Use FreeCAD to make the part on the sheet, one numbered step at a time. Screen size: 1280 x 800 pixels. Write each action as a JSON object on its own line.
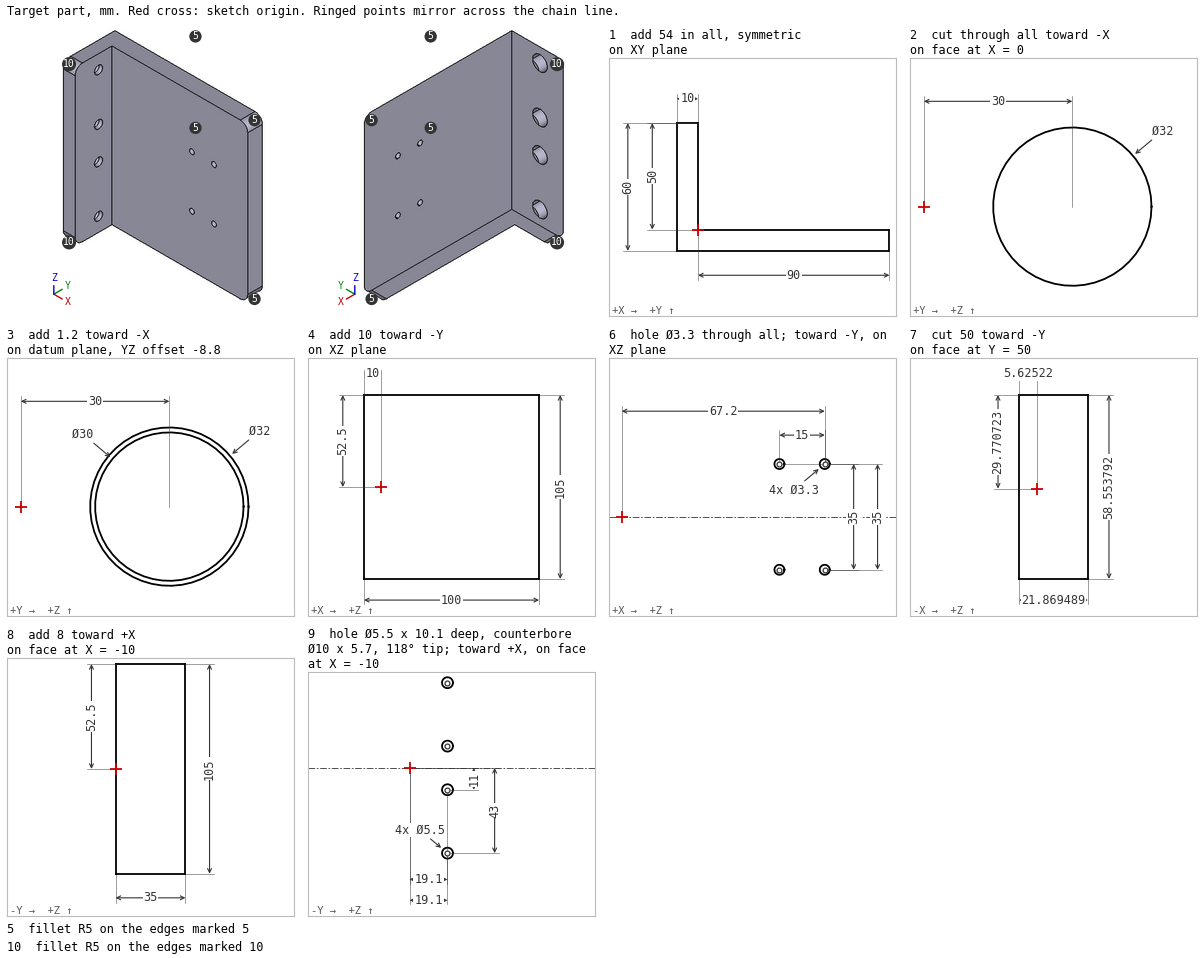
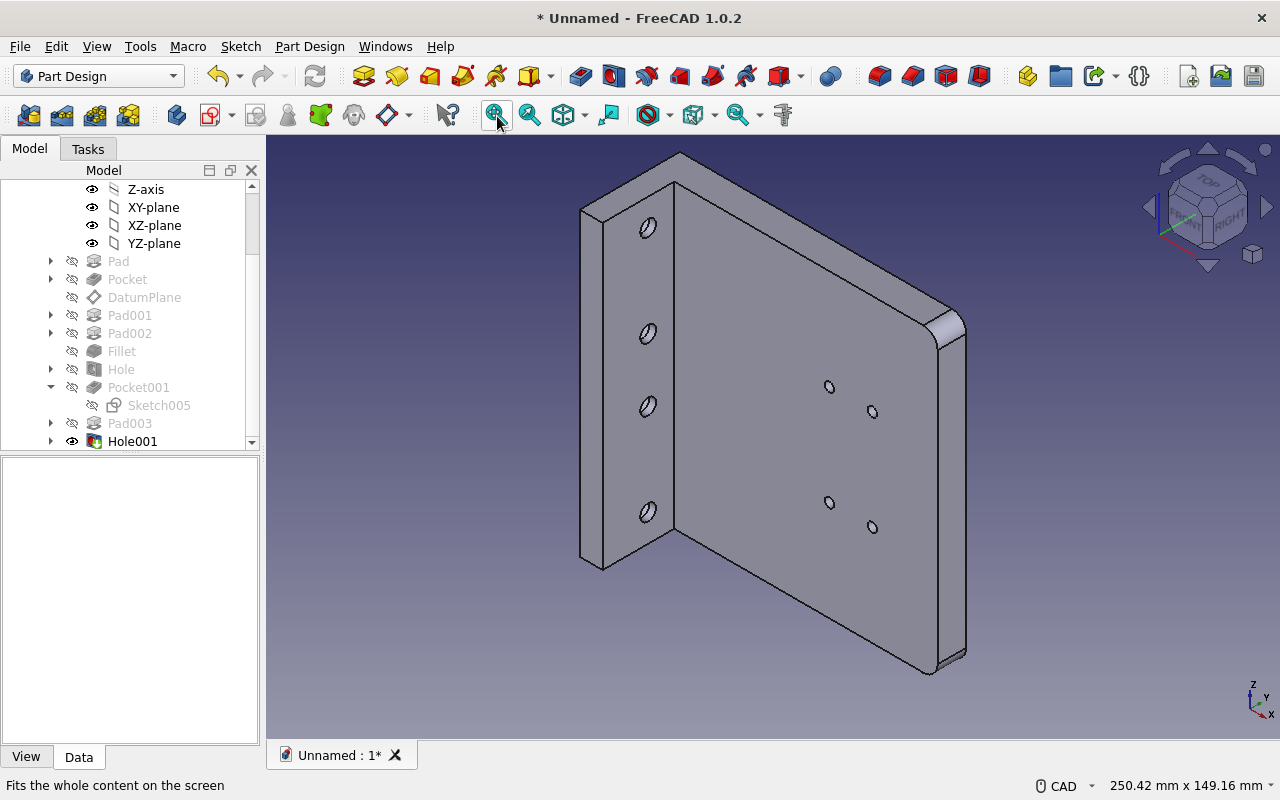
{"action": "left_click", "coordinate": [591, 215]}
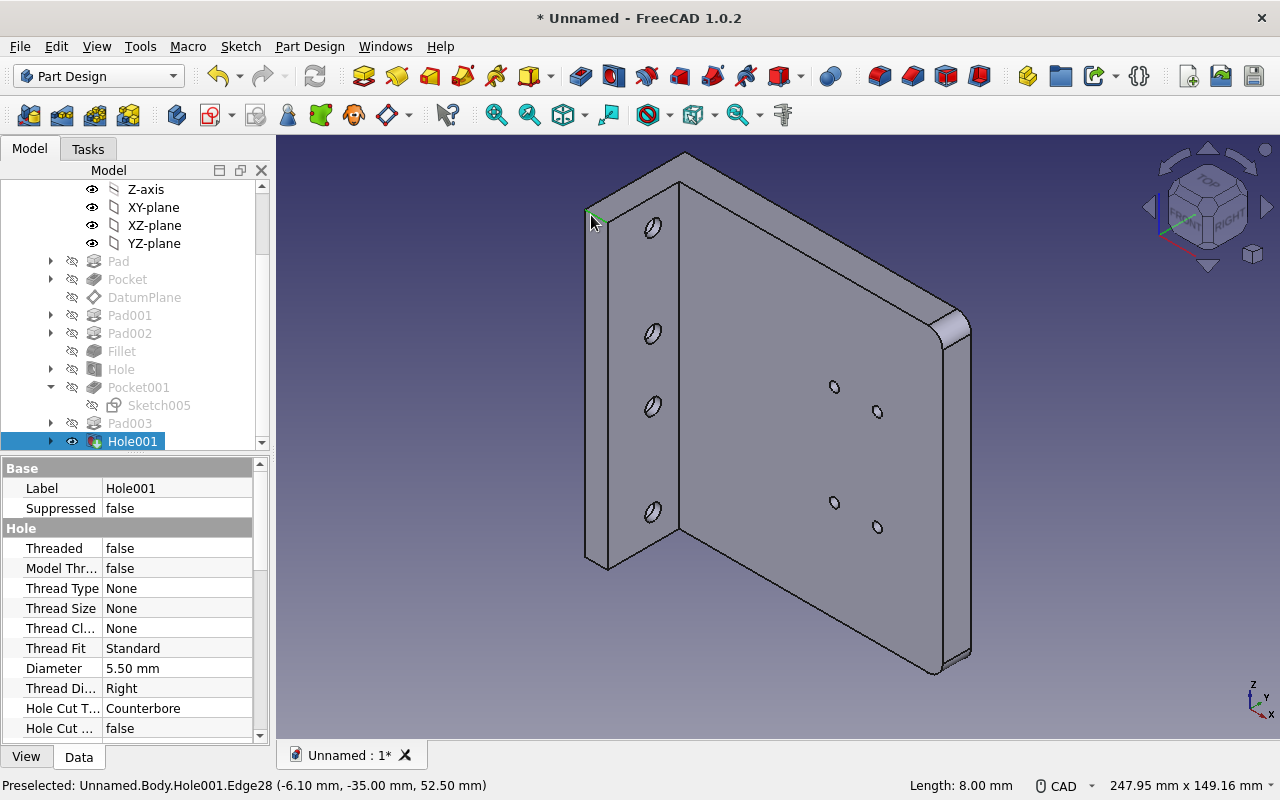
{"action": "key", "text": "2"}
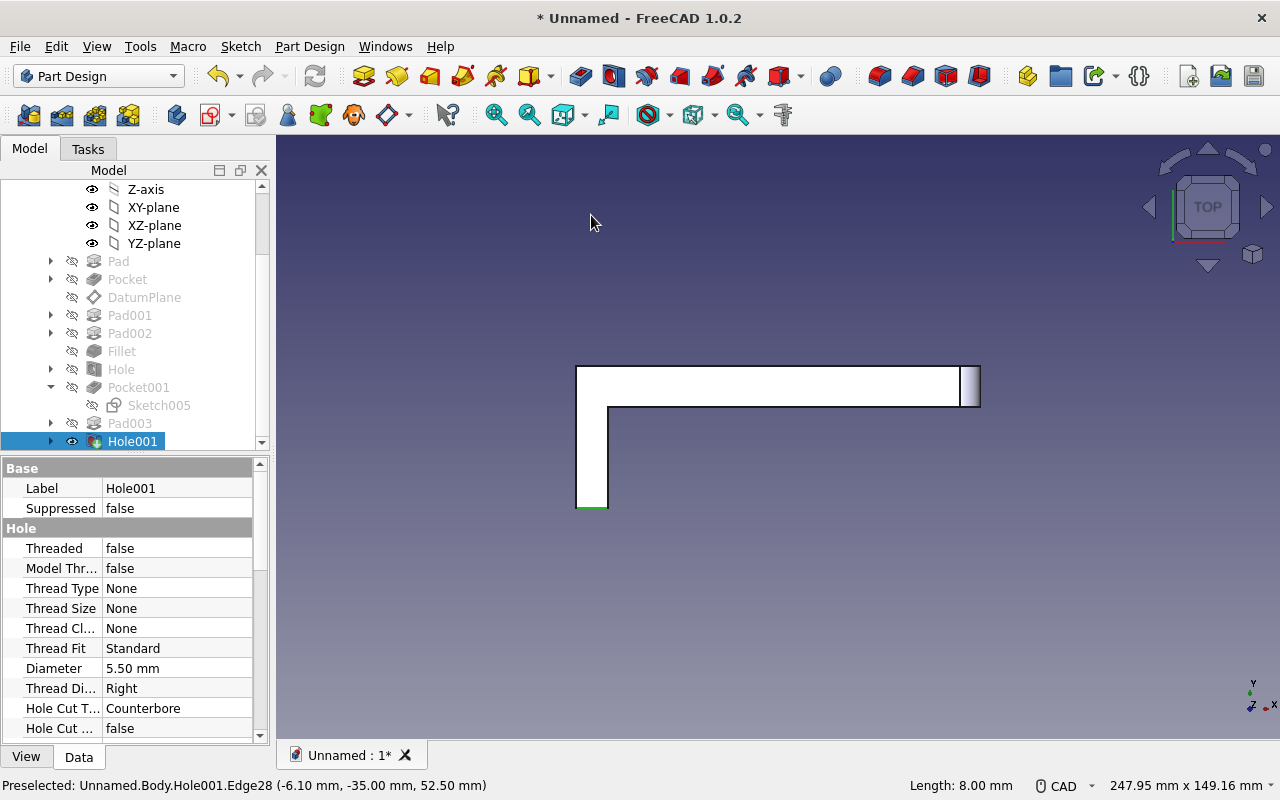
{"action": "left_click", "coordinate": [497, 116]}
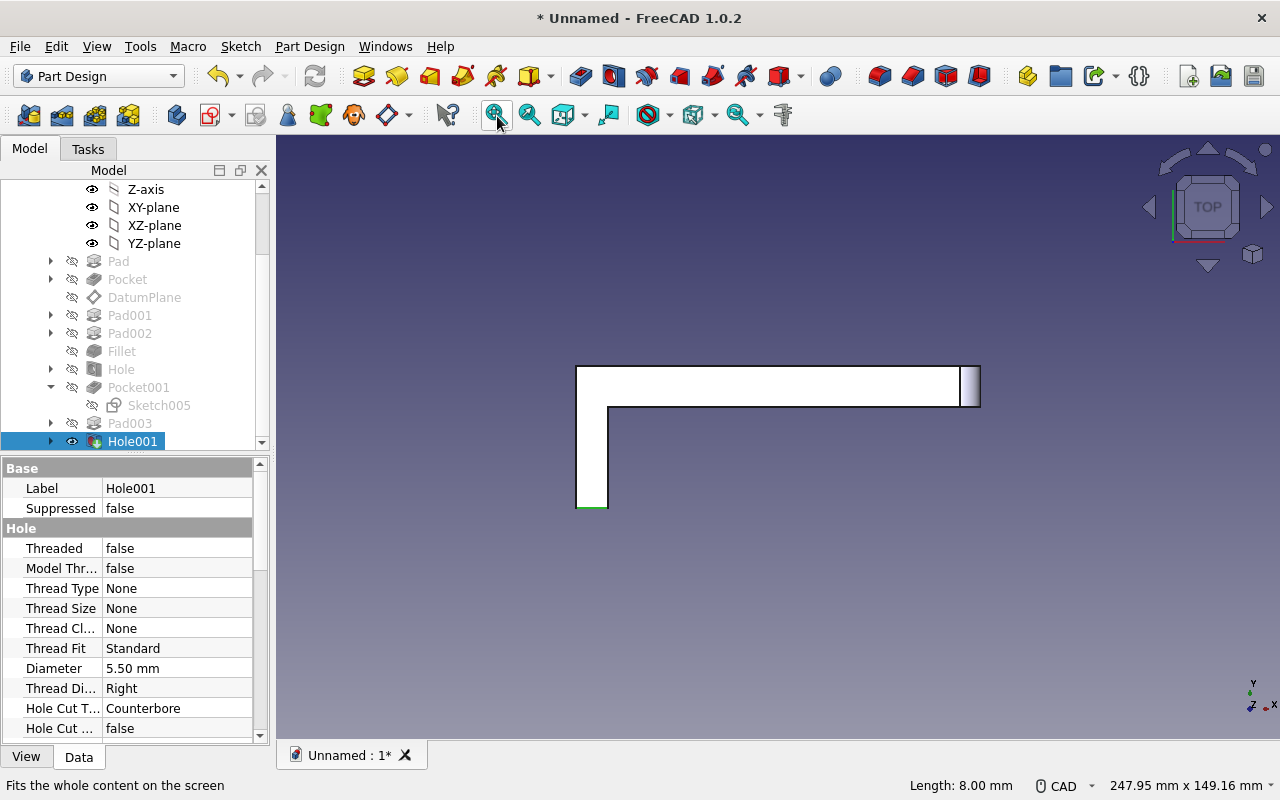
{"action": "key", "text": "1"}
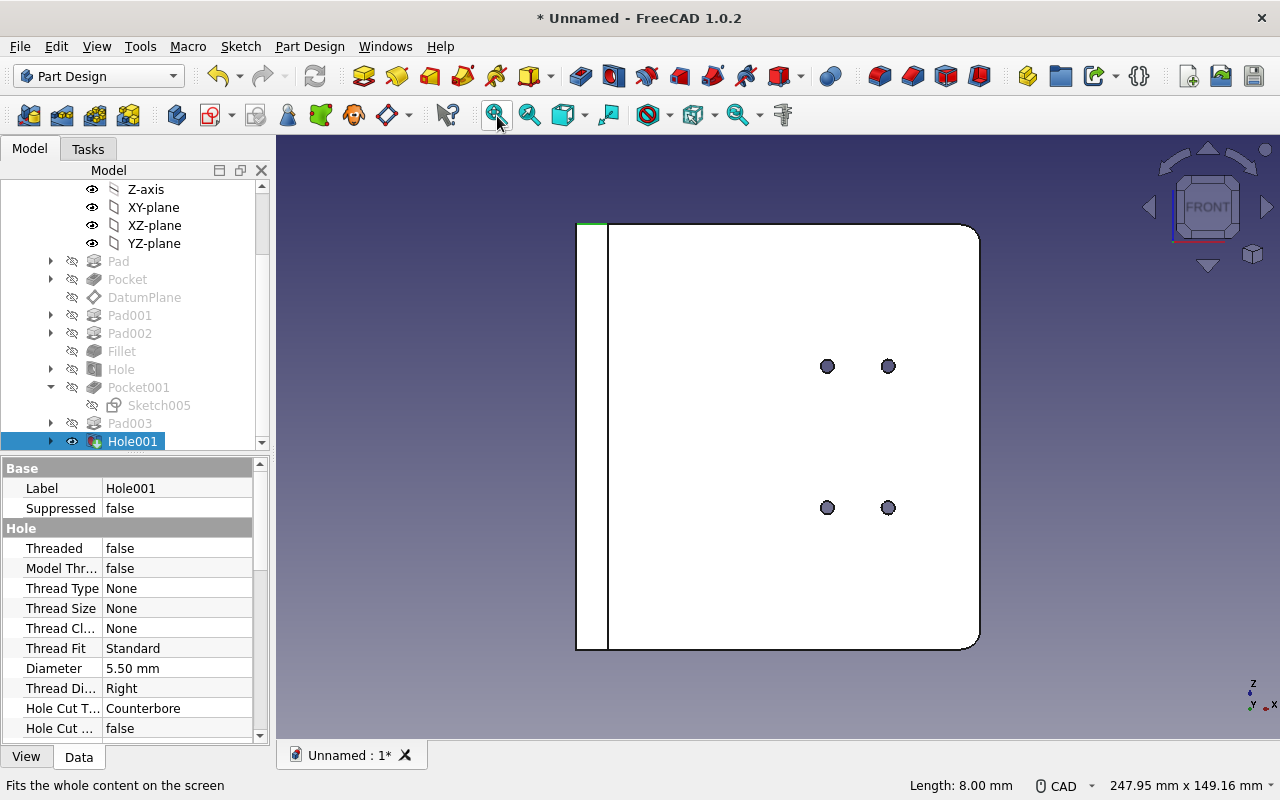
{"action": "left_click", "coordinate": [592, 649], "text": "ctrl"}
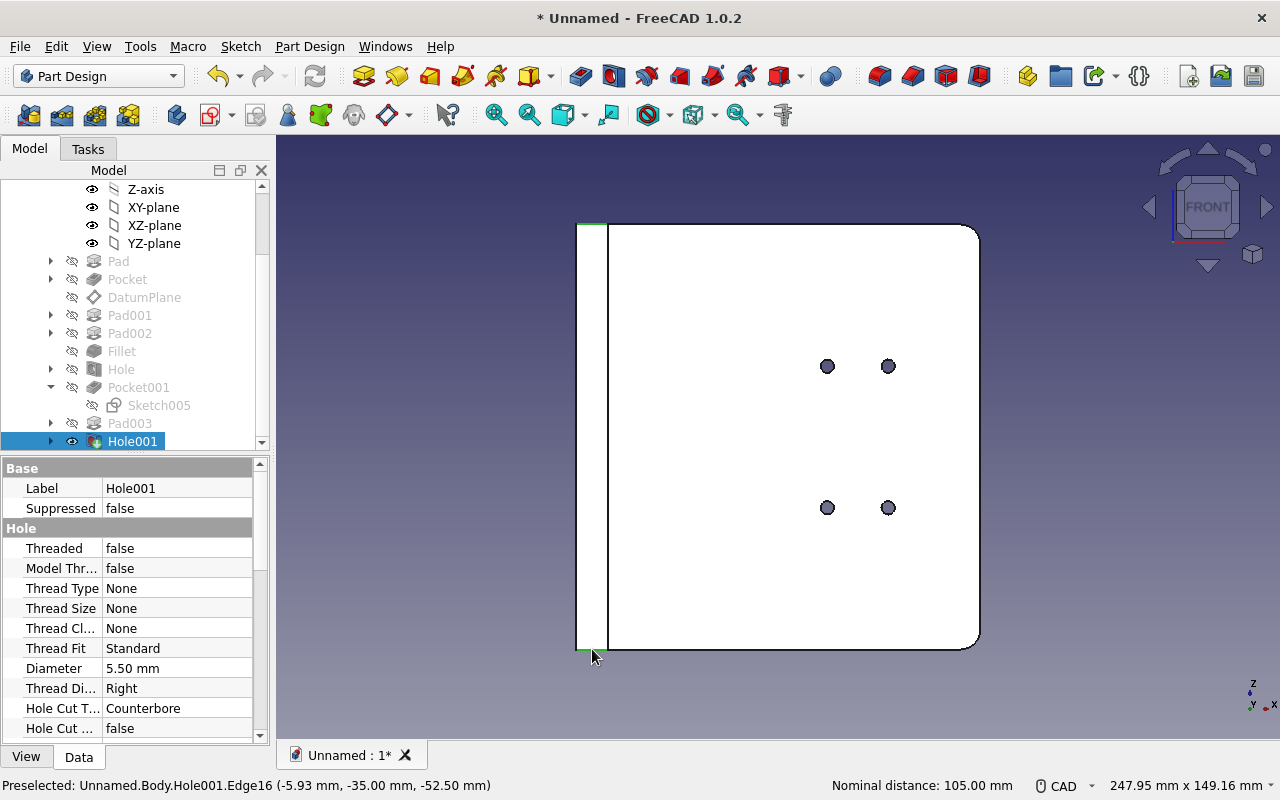
{"action": "left_click", "coordinate": [880, 76]}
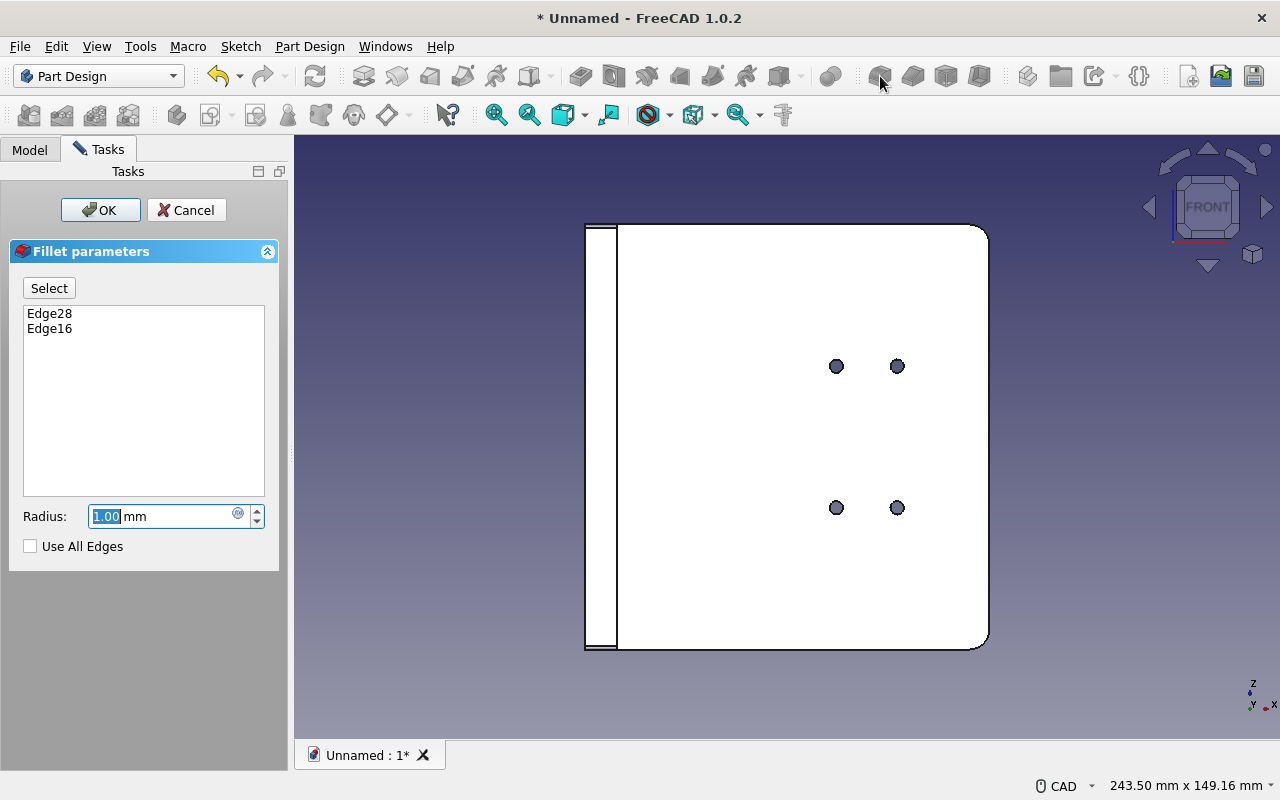
{"action": "type", "text": "5"}
{"action": "key", "text": "Tab"}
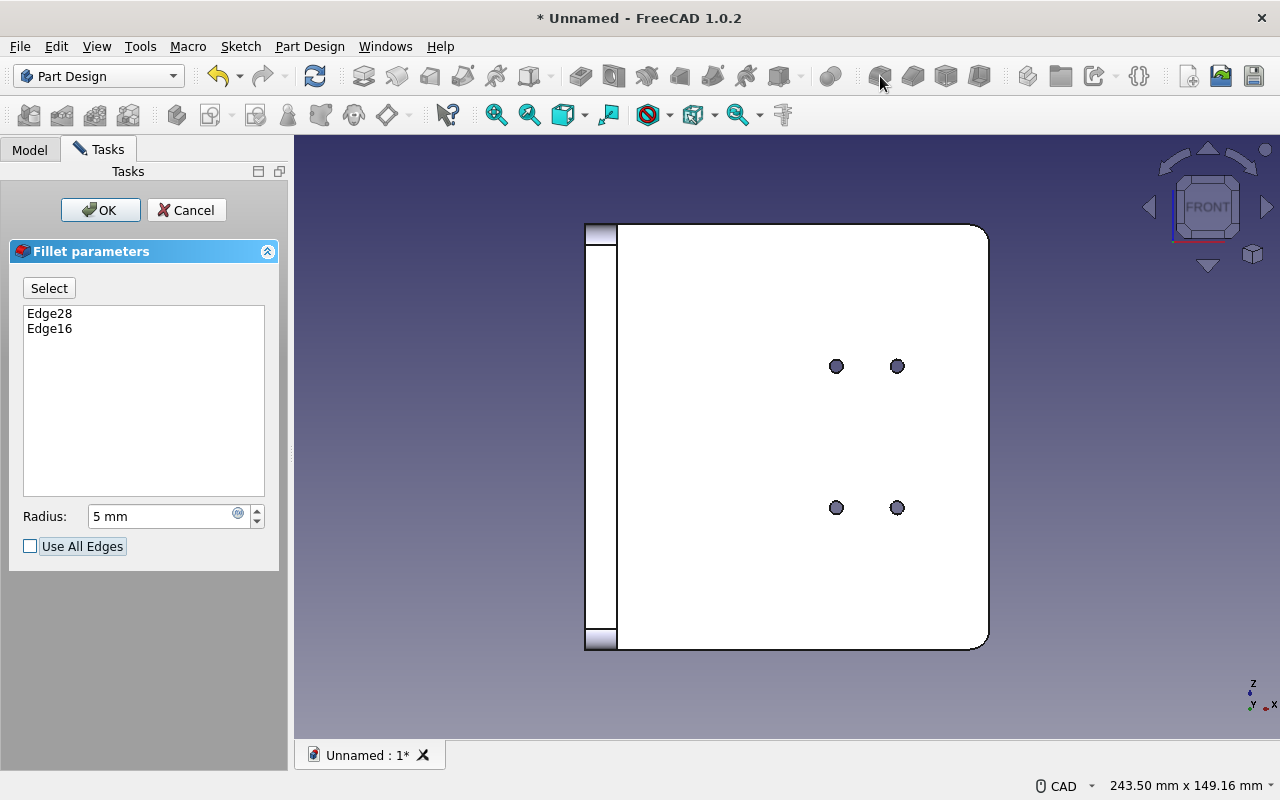
{"action": "left_click", "coordinate": [101, 210]}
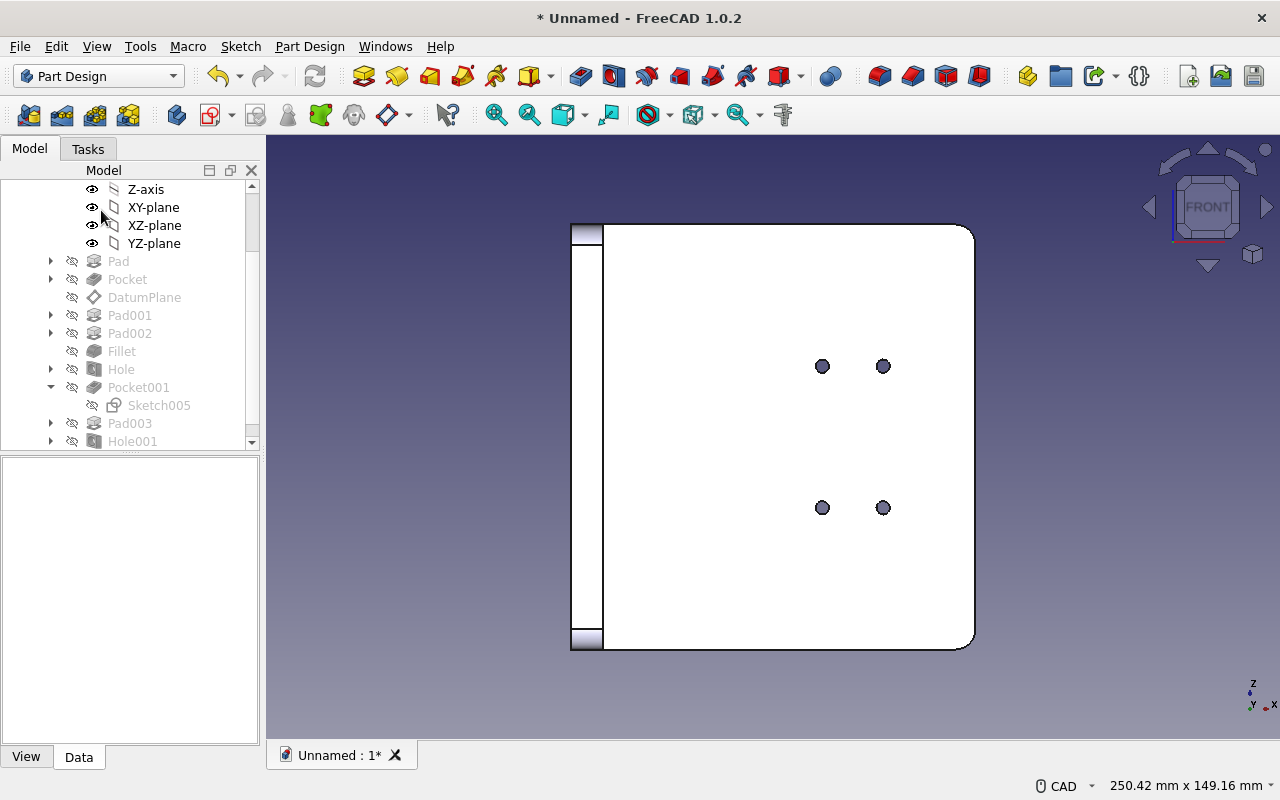
{"action": "key", "text": "0"}